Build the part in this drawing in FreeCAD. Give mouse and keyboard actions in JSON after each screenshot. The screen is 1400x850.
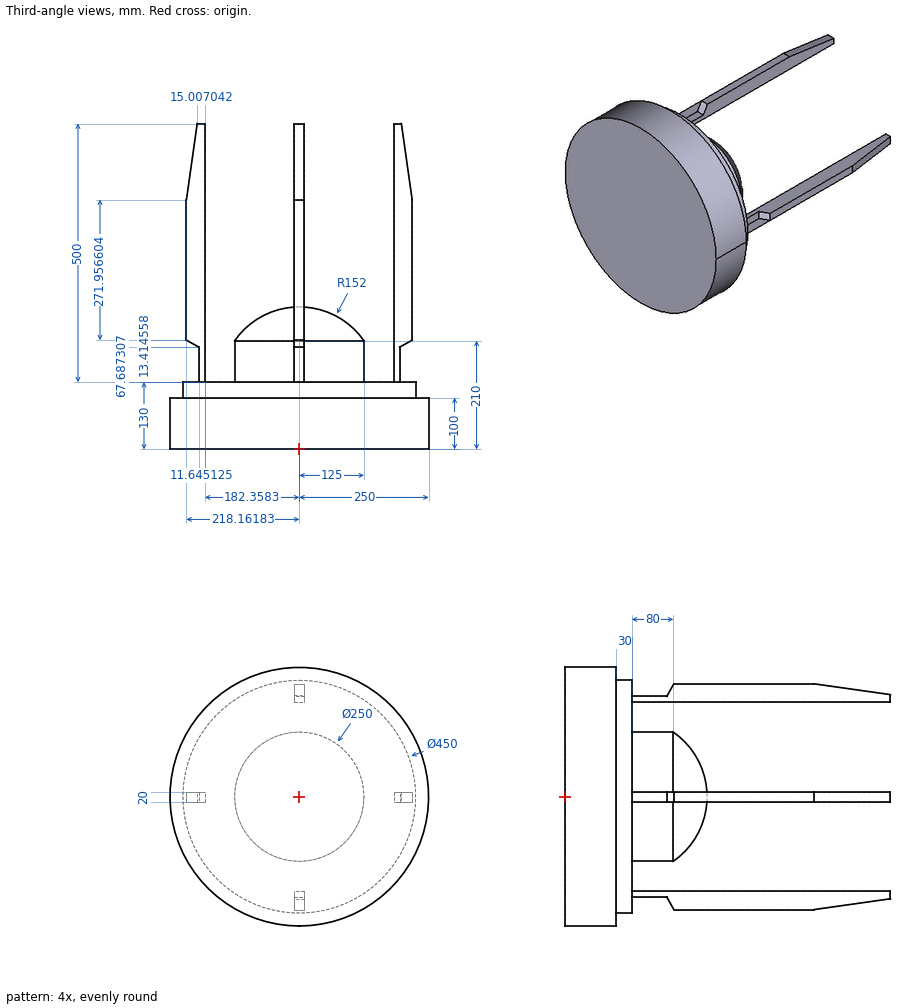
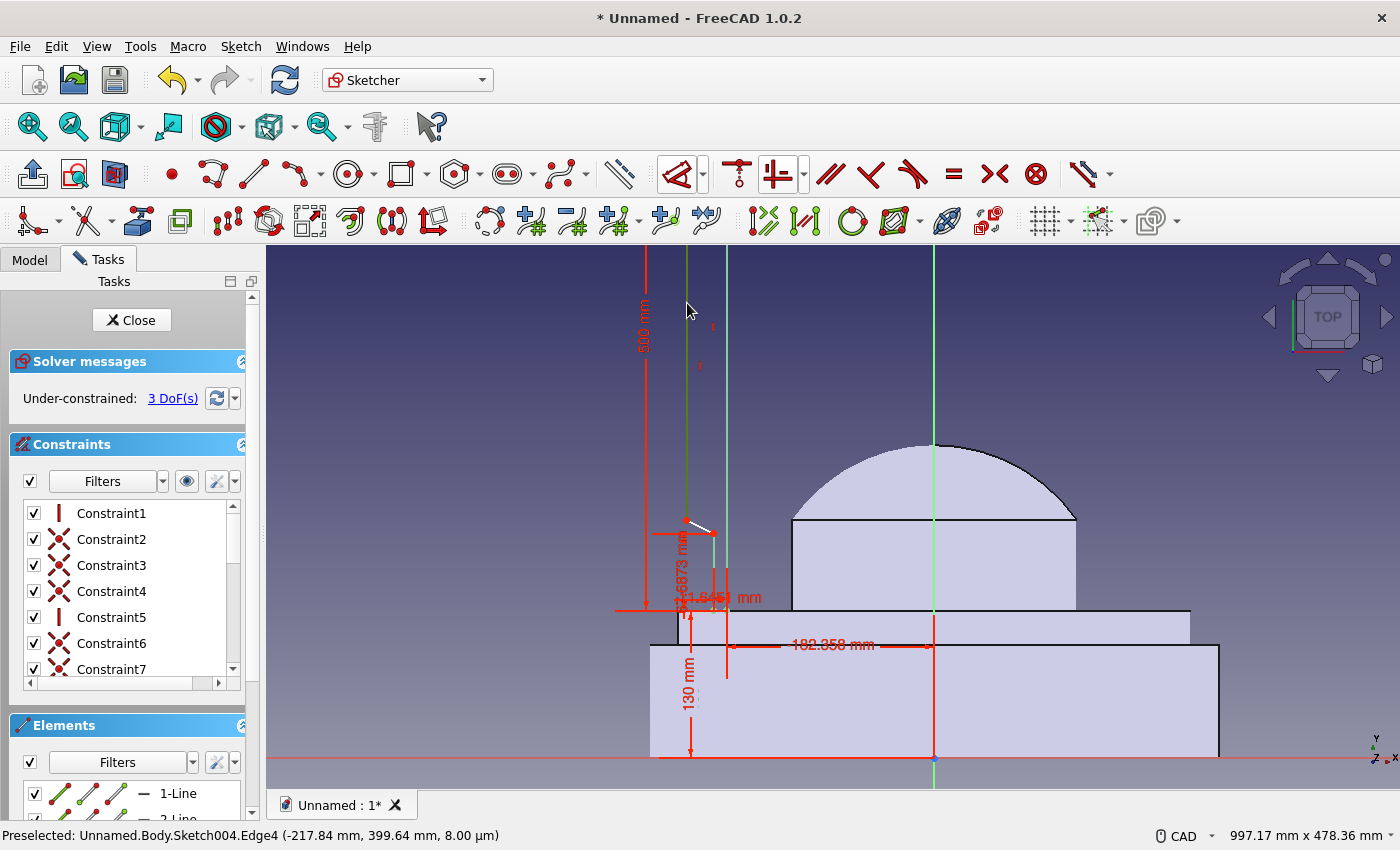
{"action": "key", "text": "i"}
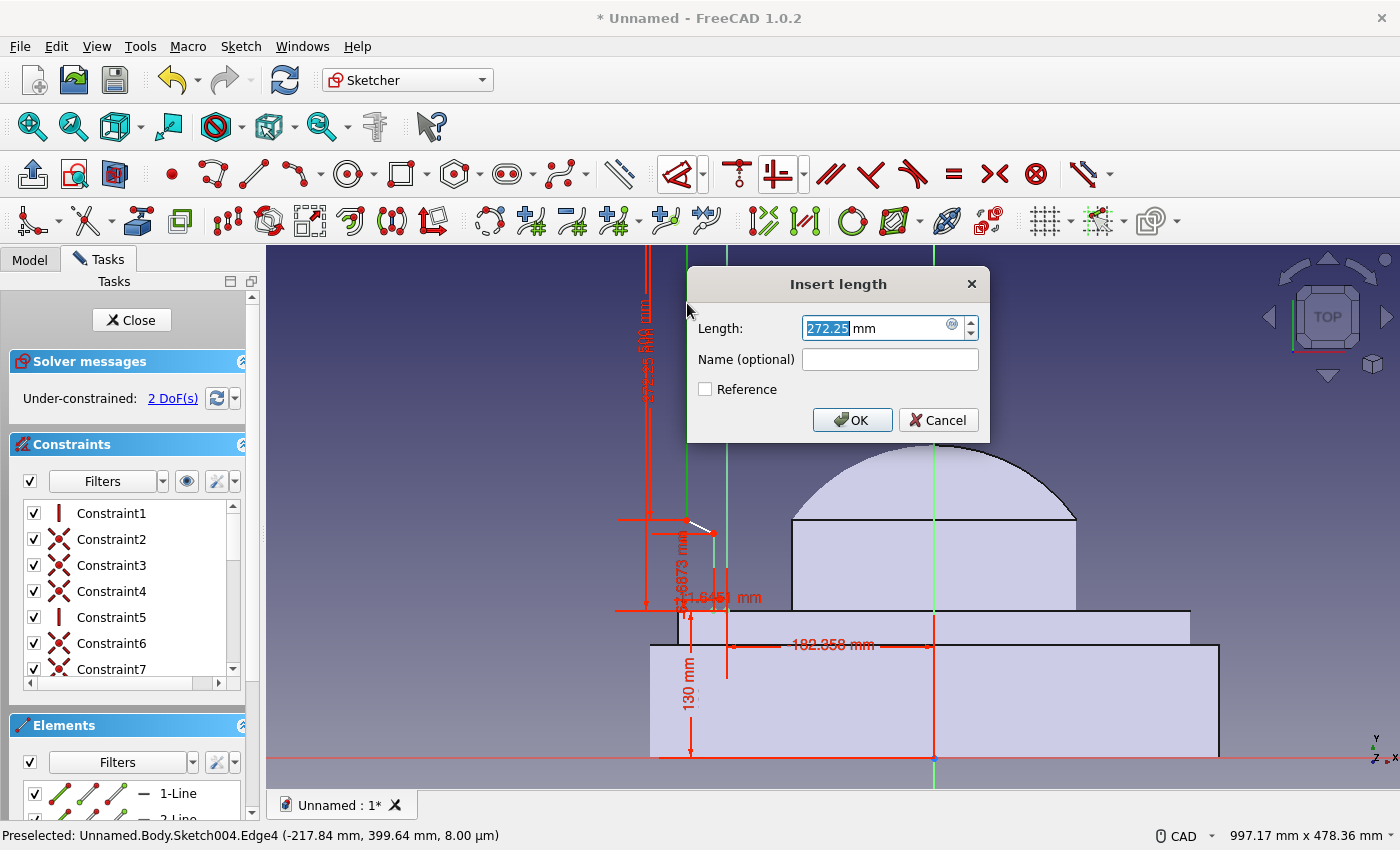
{"action": "type", "text": "271.956604"}
{"action": "key", "text": "Return"}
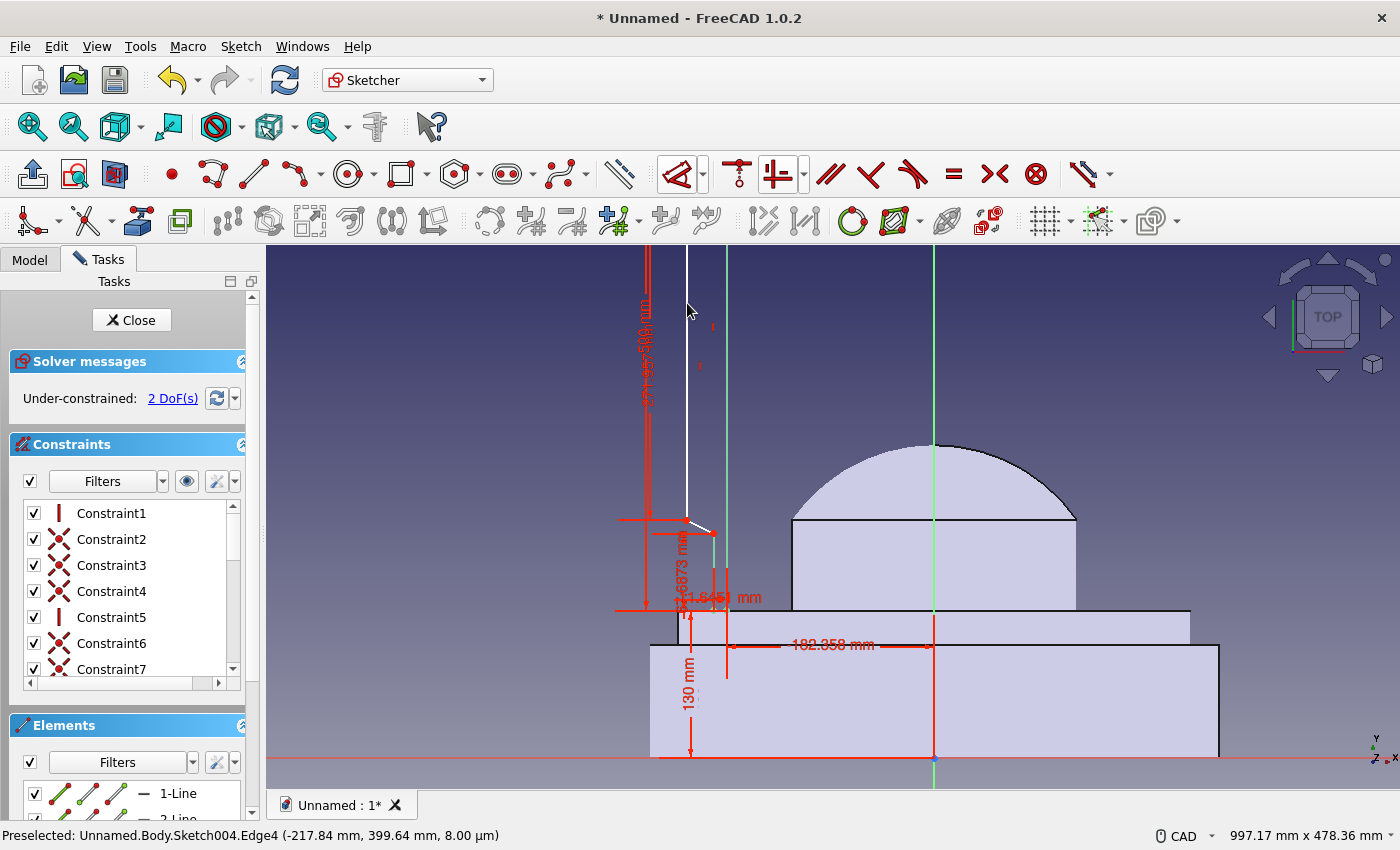
{"action": "scroll", "coordinate": [727, 612], "scroll_direction": "down", "scroll_amount": 4}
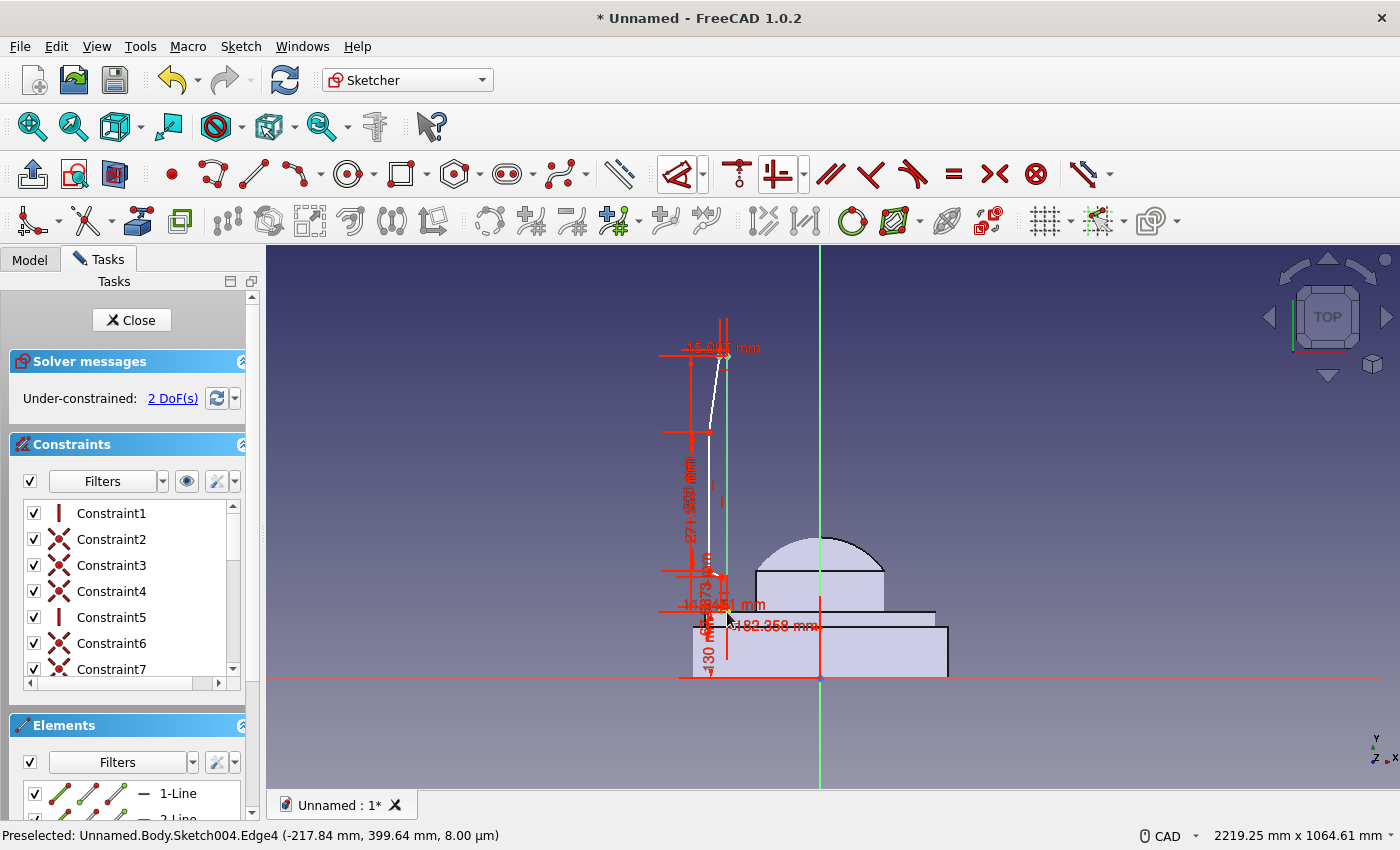
{"action": "left_click", "coordinate": [709, 432]}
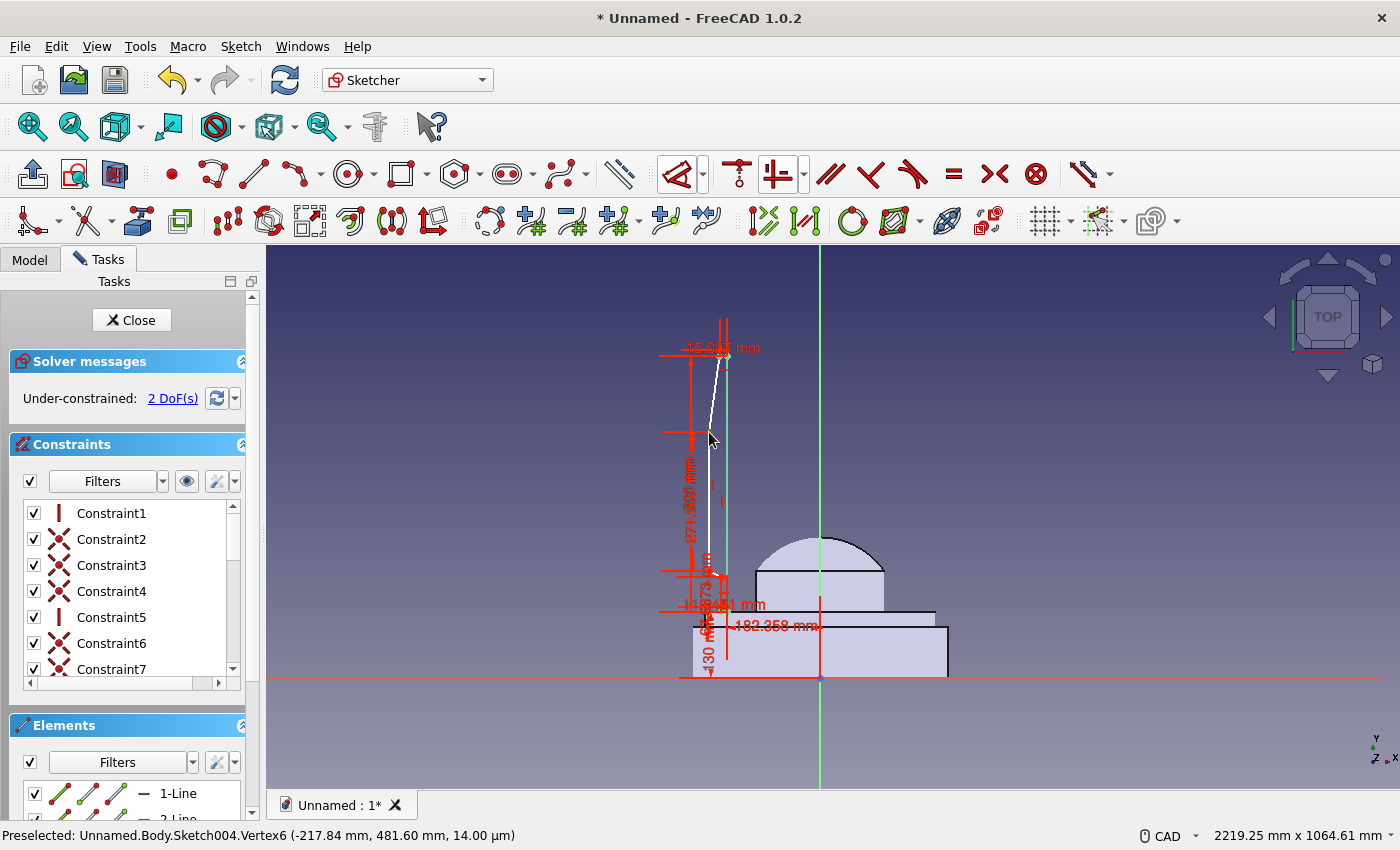
{"action": "left_click", "coordinate": [702, 174]}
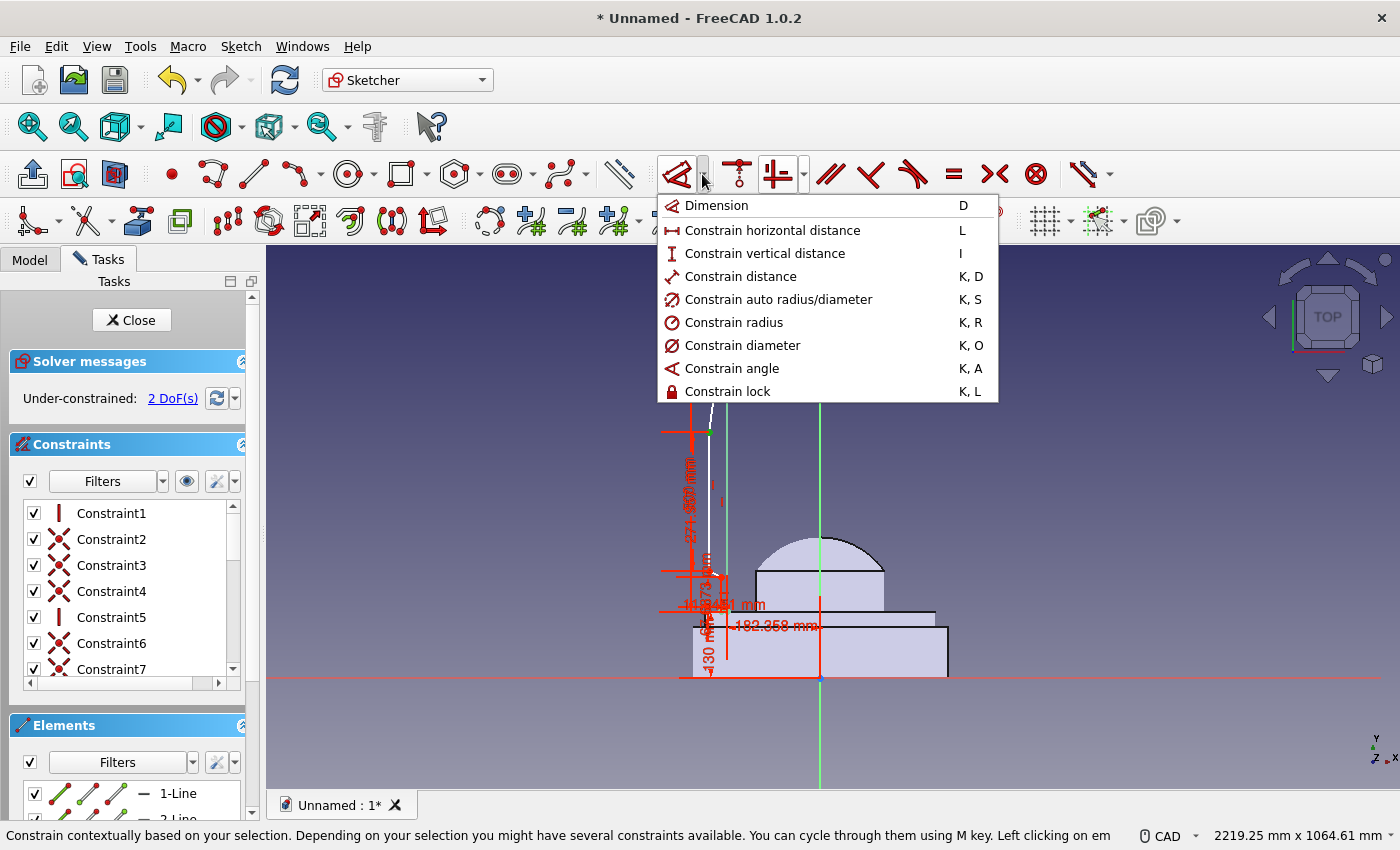
{"action": "left_click", "coordinate": [828, 230]}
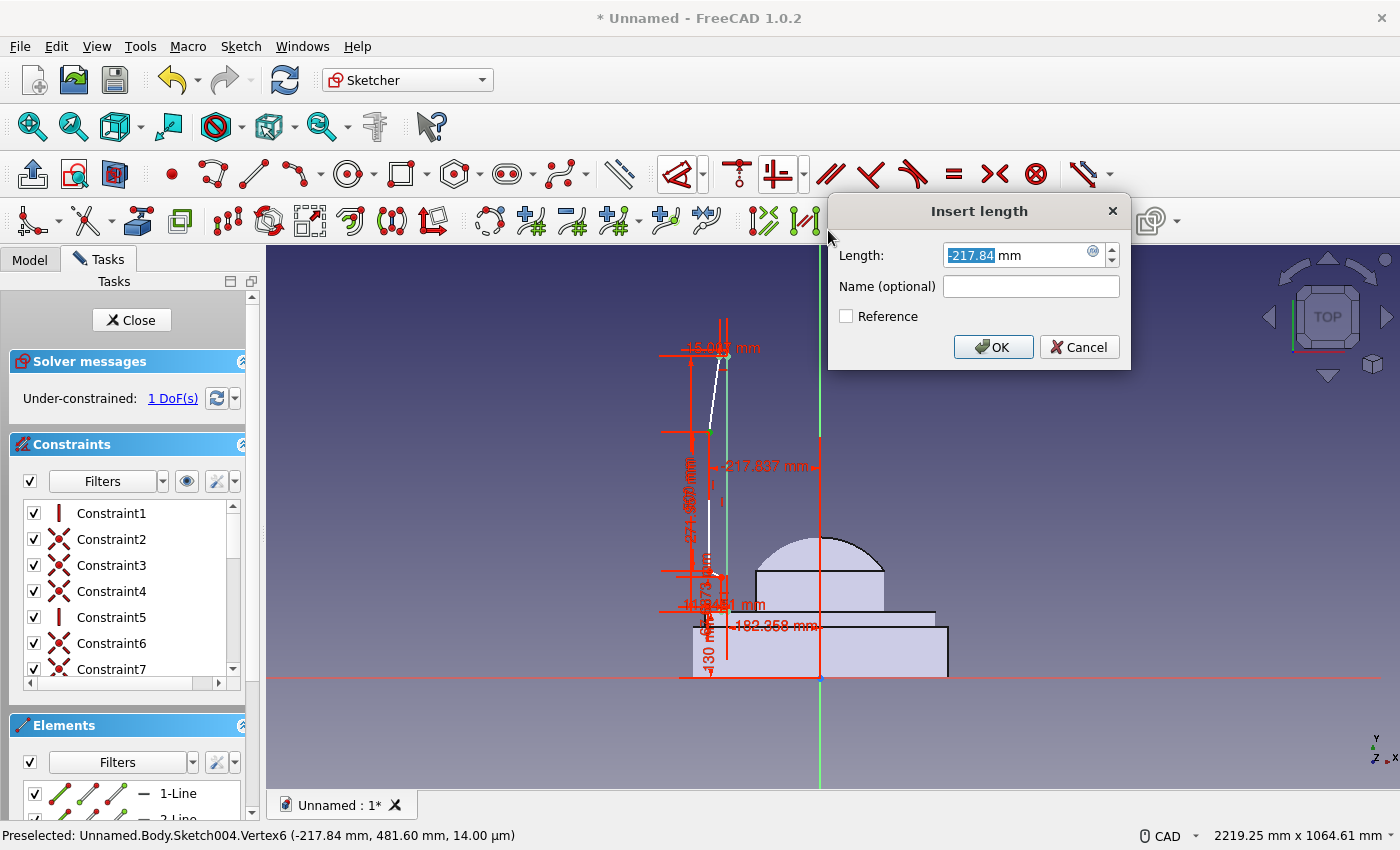
{"action": "type", "text": "-218.16183"}
{"action": "key", "text": "Return"}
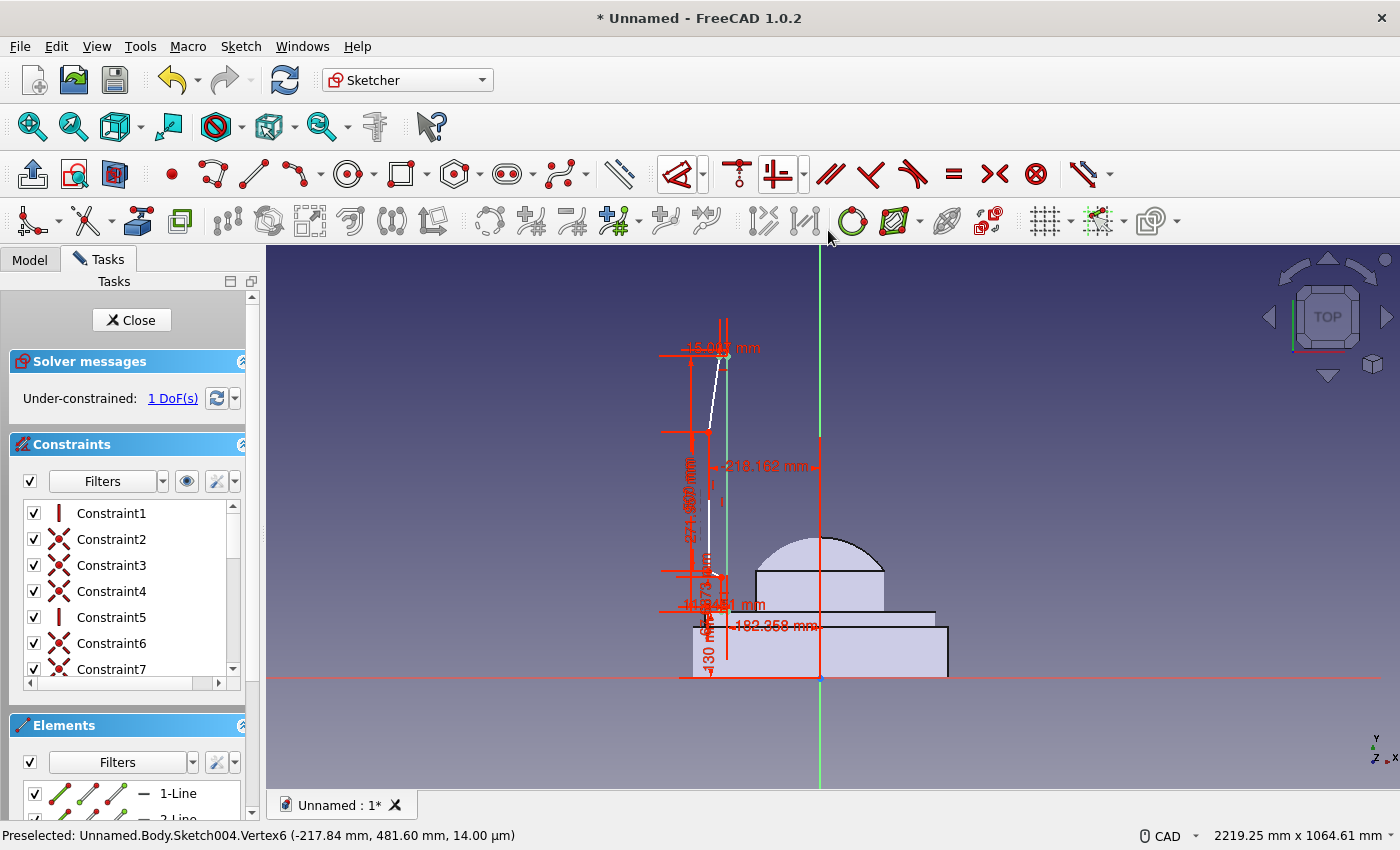
{"action": "scroll", "coordinate": [715, 574], "scroll_direction": "up", "scroll_amount": 9}